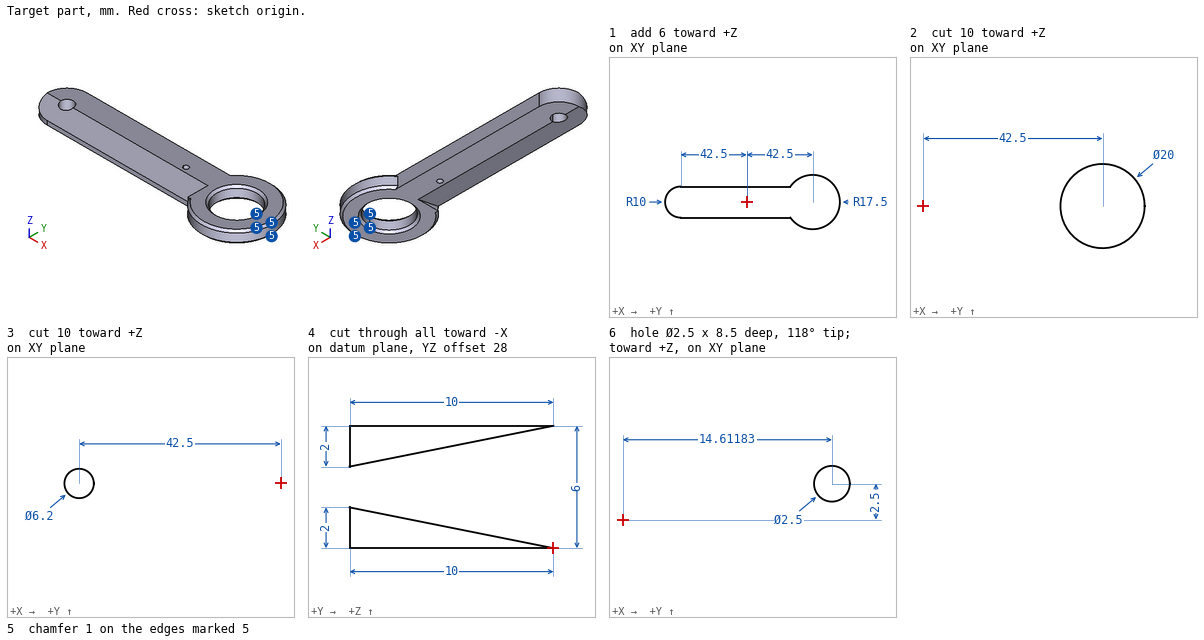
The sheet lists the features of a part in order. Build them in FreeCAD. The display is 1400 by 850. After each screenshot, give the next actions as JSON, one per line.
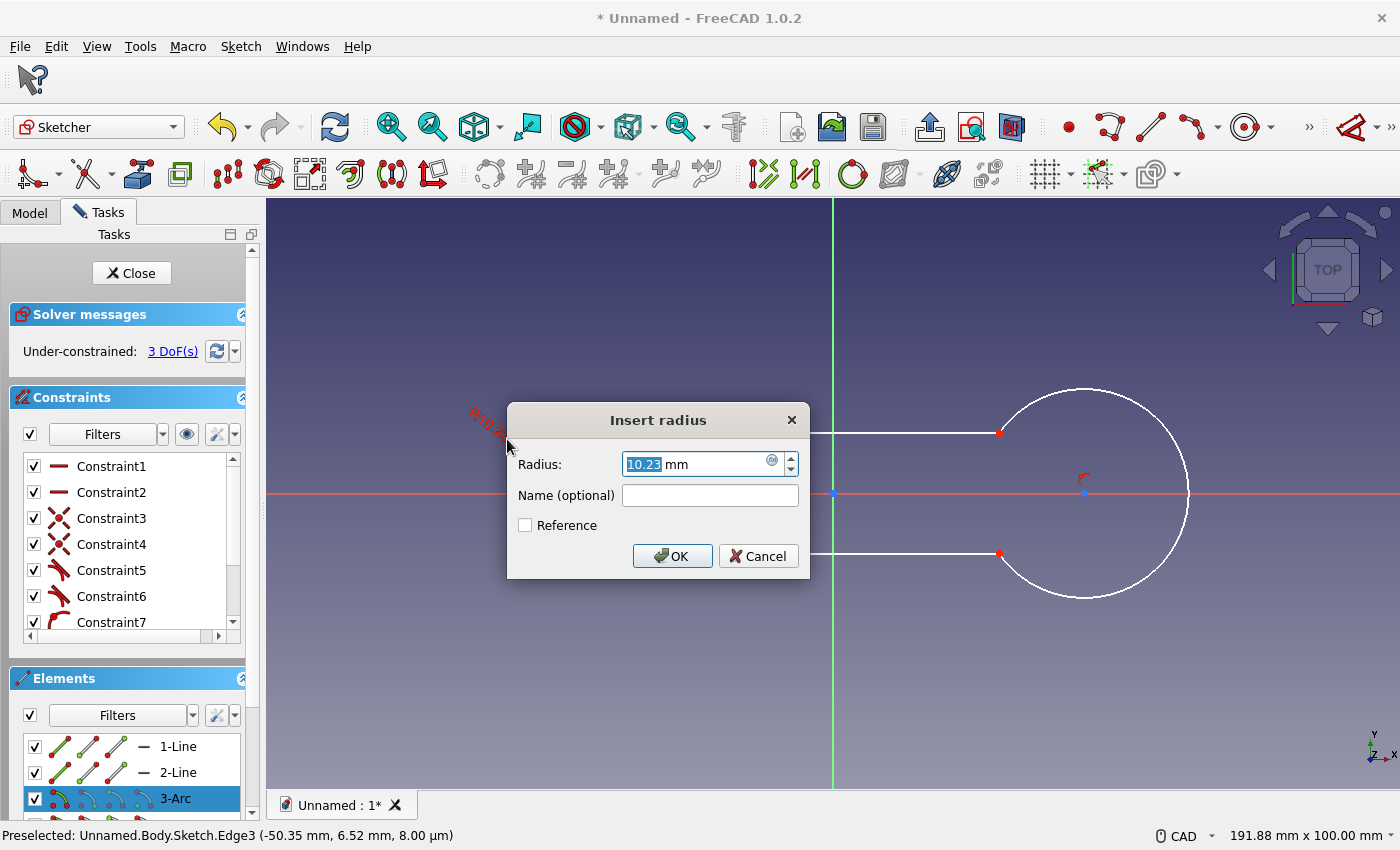
{"action": "type", "text": "10"}
{"action": "key", "text": "Return"}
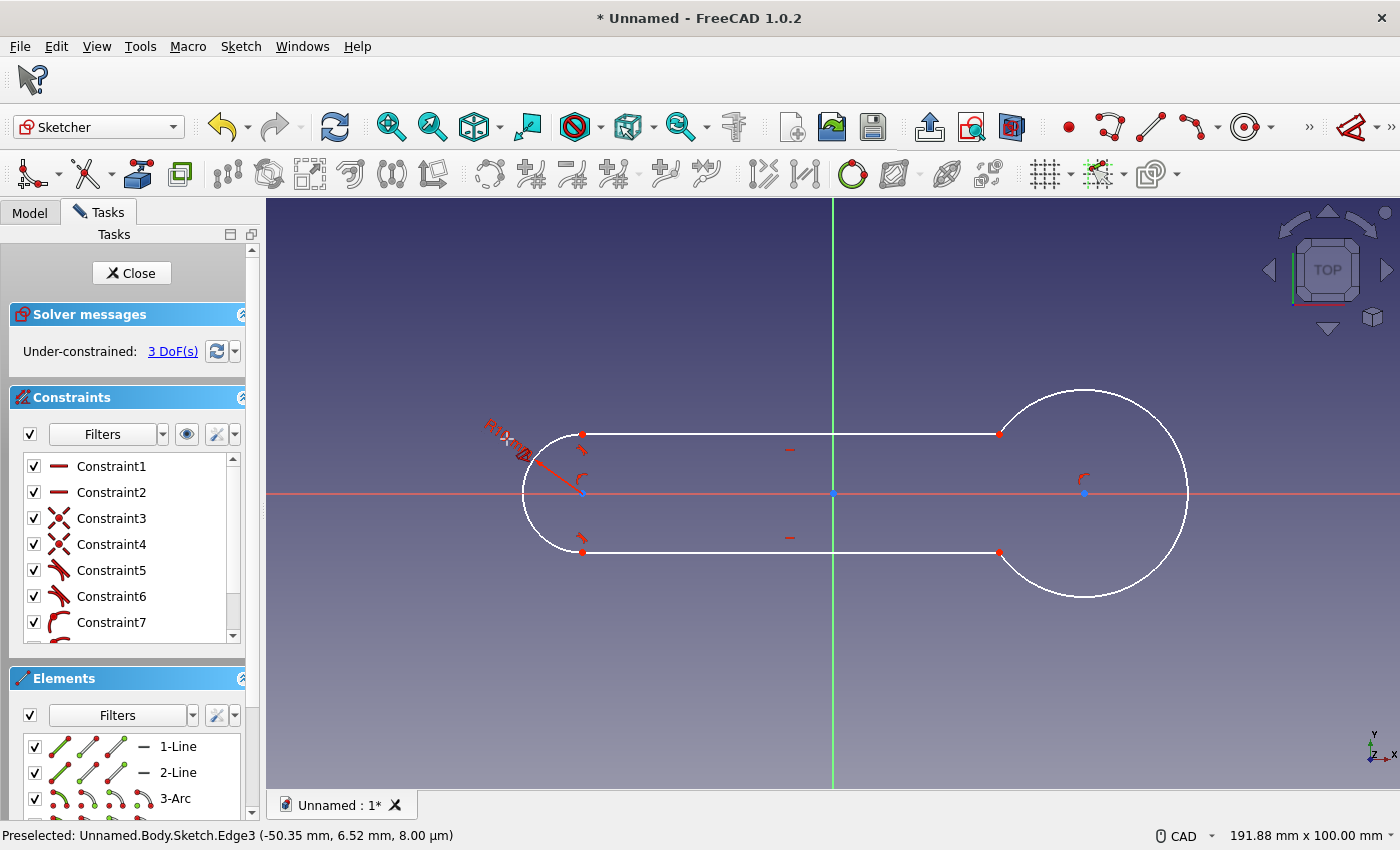
{"action": "left_click", "coordinate": [1139, 582]}
{"action": "left_click", "coordinate": [1156, 609]}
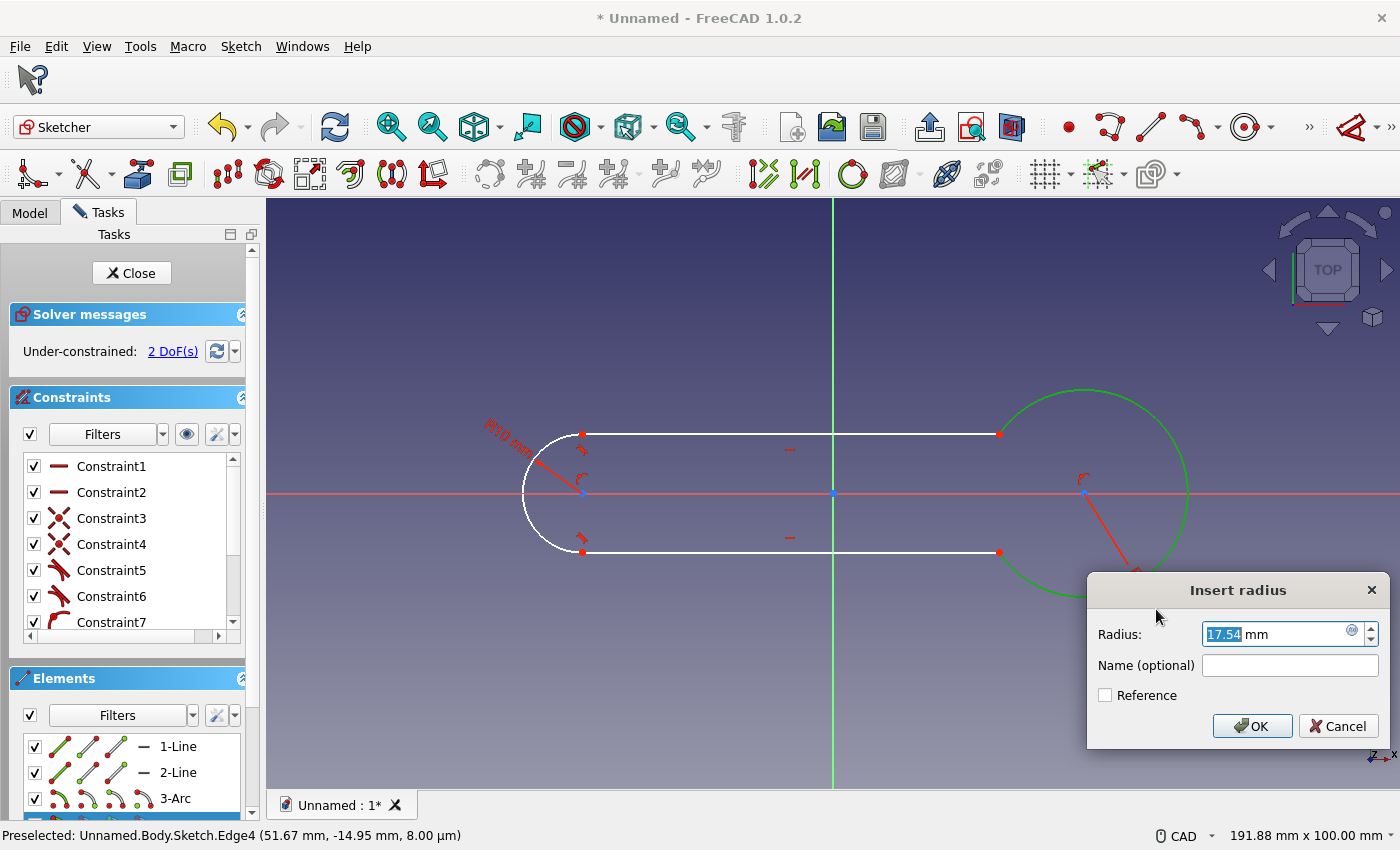
{"action": "type", "text": "17.5"}
{"action": "key", "text": "Return"}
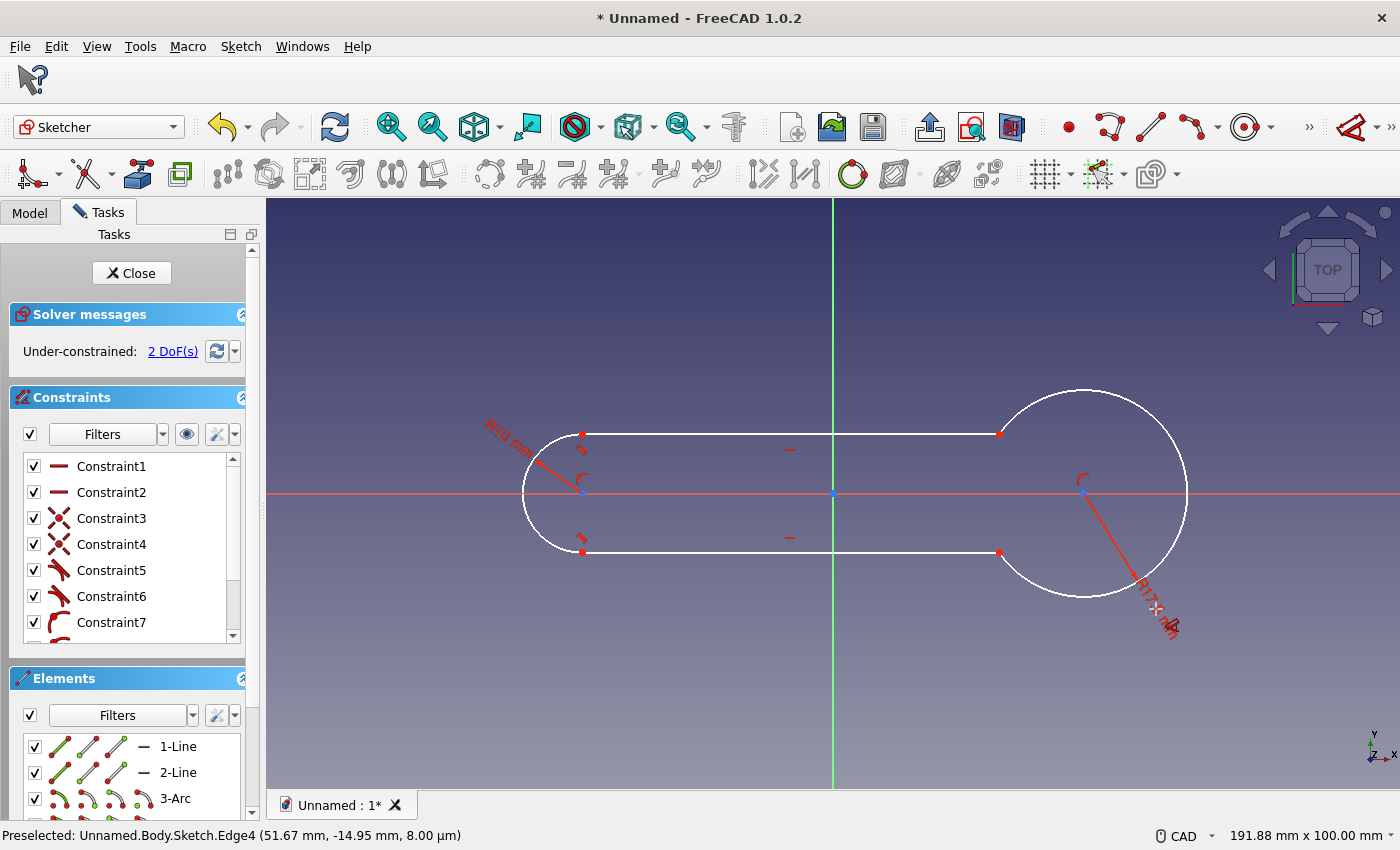
{"action": "left_click", "coordinate": [582, 434]}
{"action": "left_click", "coordinate": [708, 400]}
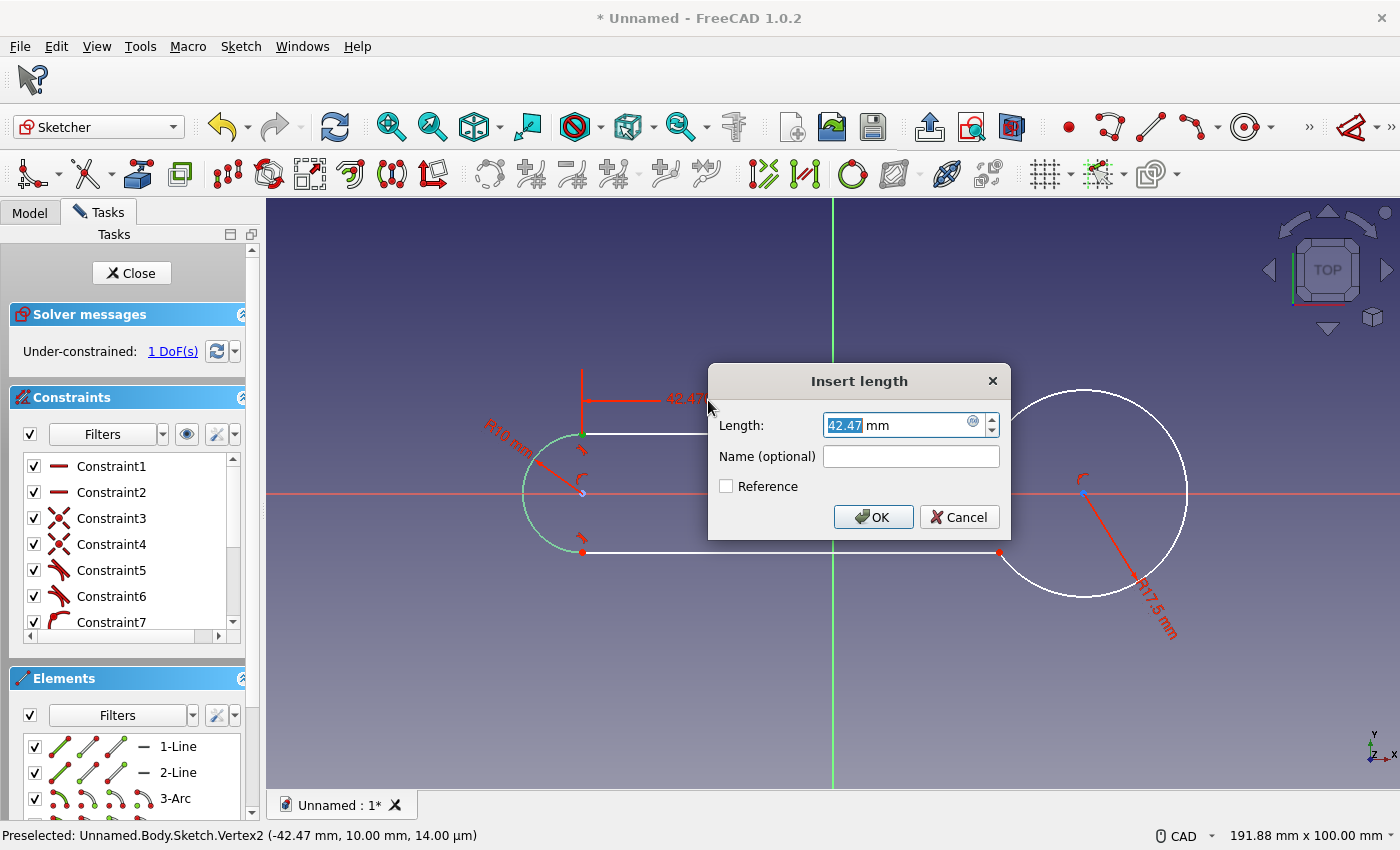
{"action": "type", "text": "42.5"}
{"action": "key", "text": "Return"}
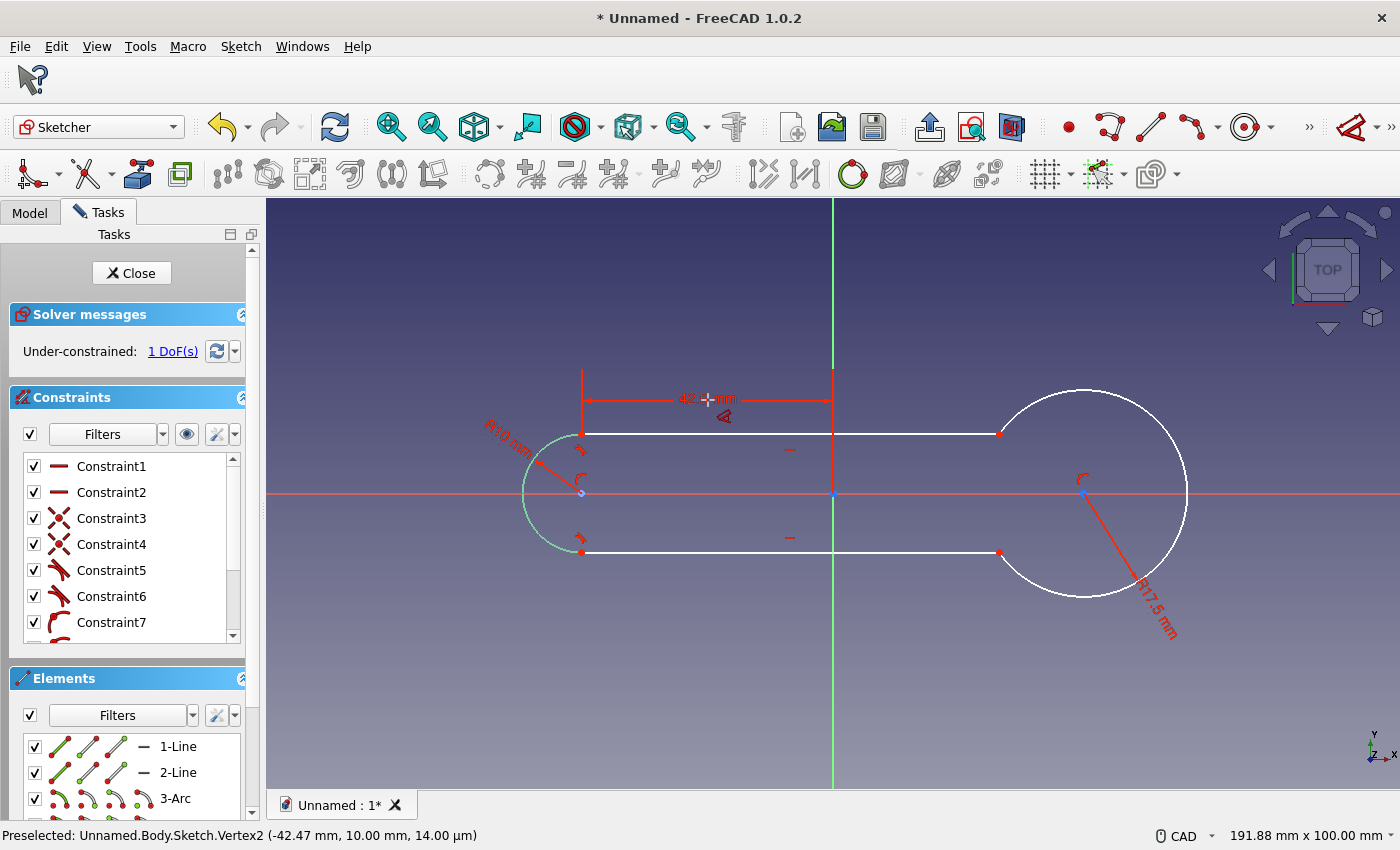
{"action": "left_click", "coordinate": [1084, 494]}
{"action": "left_click", "coordinate": [958, 528]}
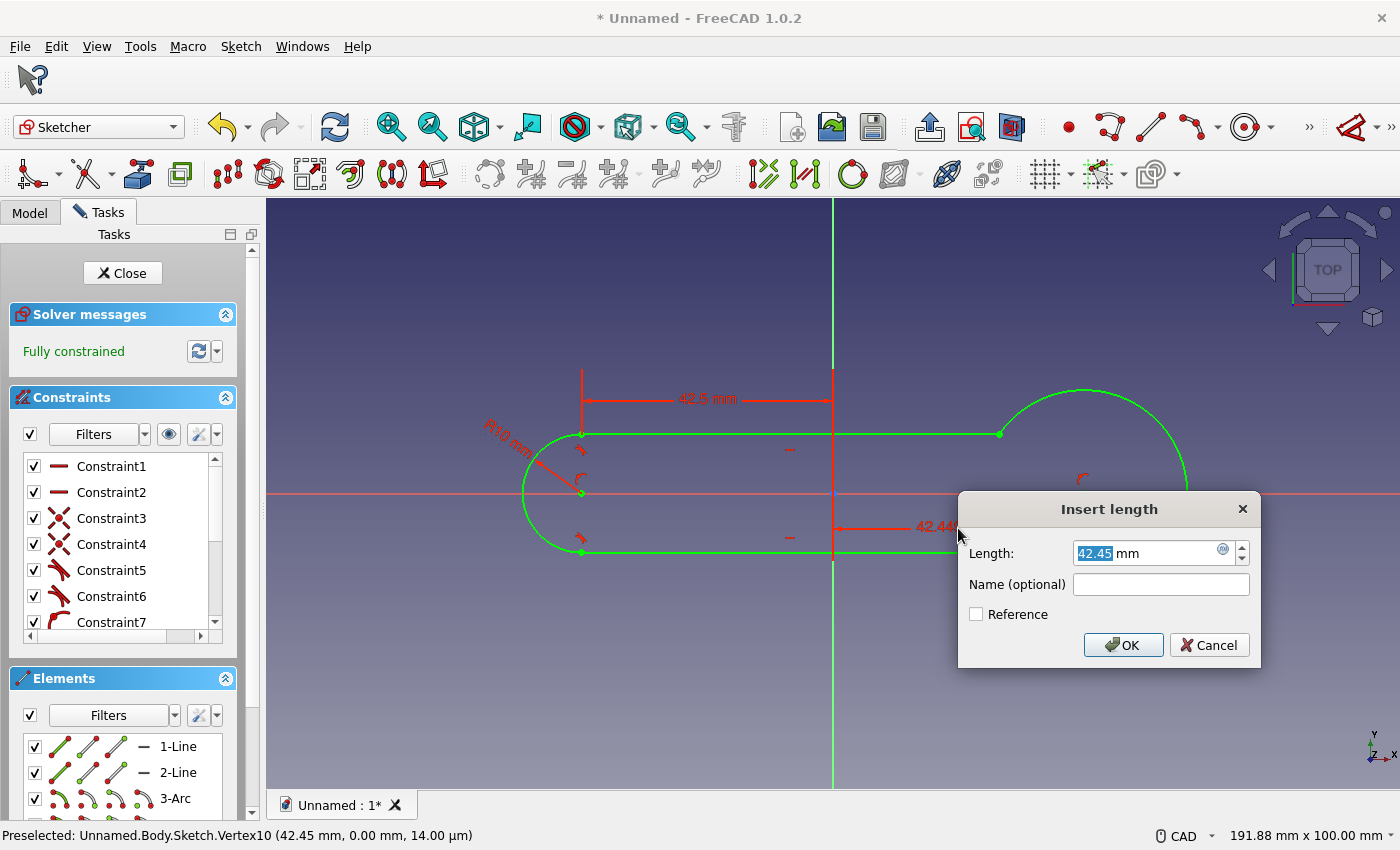
{"action": "type", "text": "42.5"}
{"action": "key", "text": "Return"}
{"action": "key", "text": "Escape"}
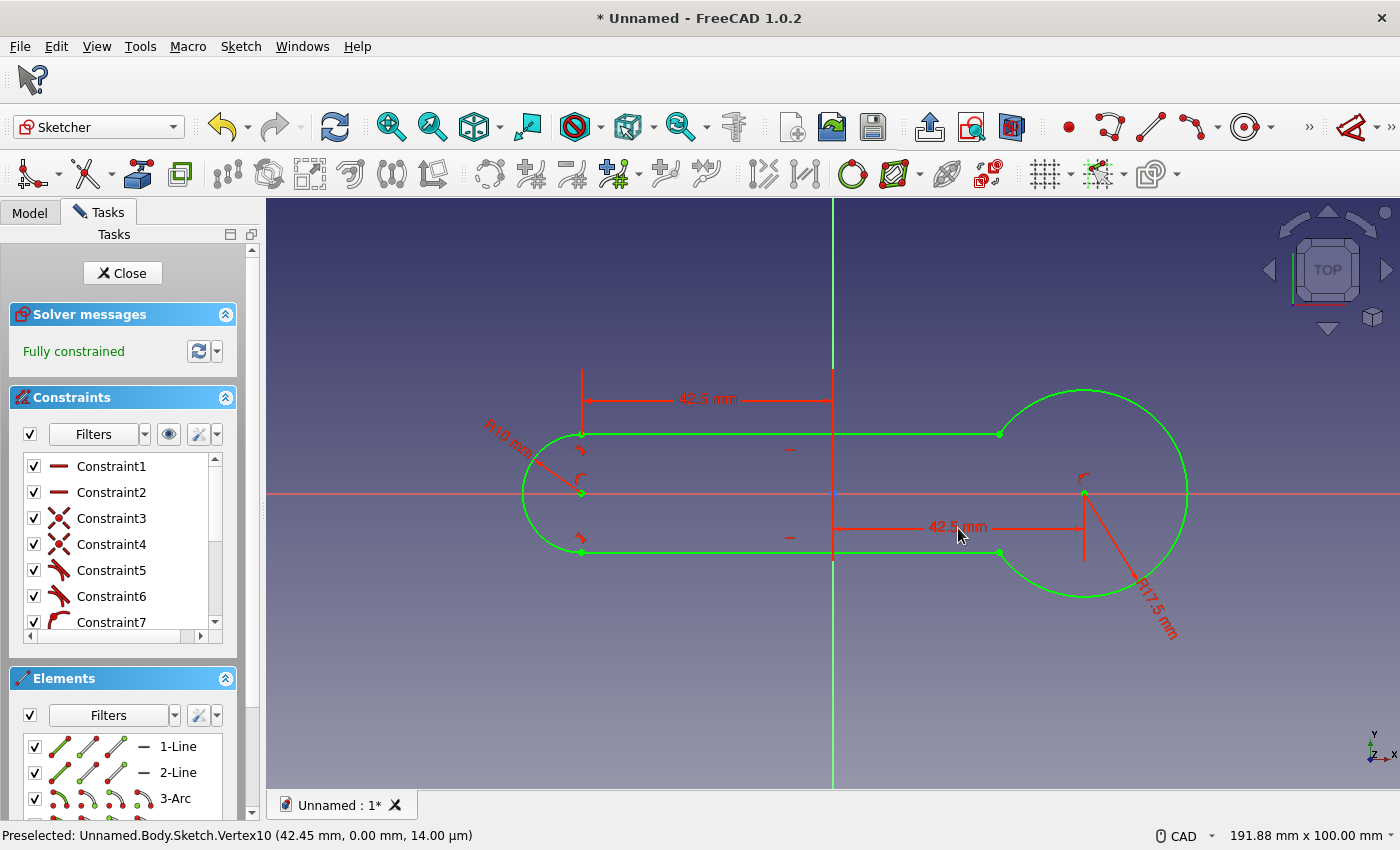
{"action": "left_click", "coordinate": [123, 273]}